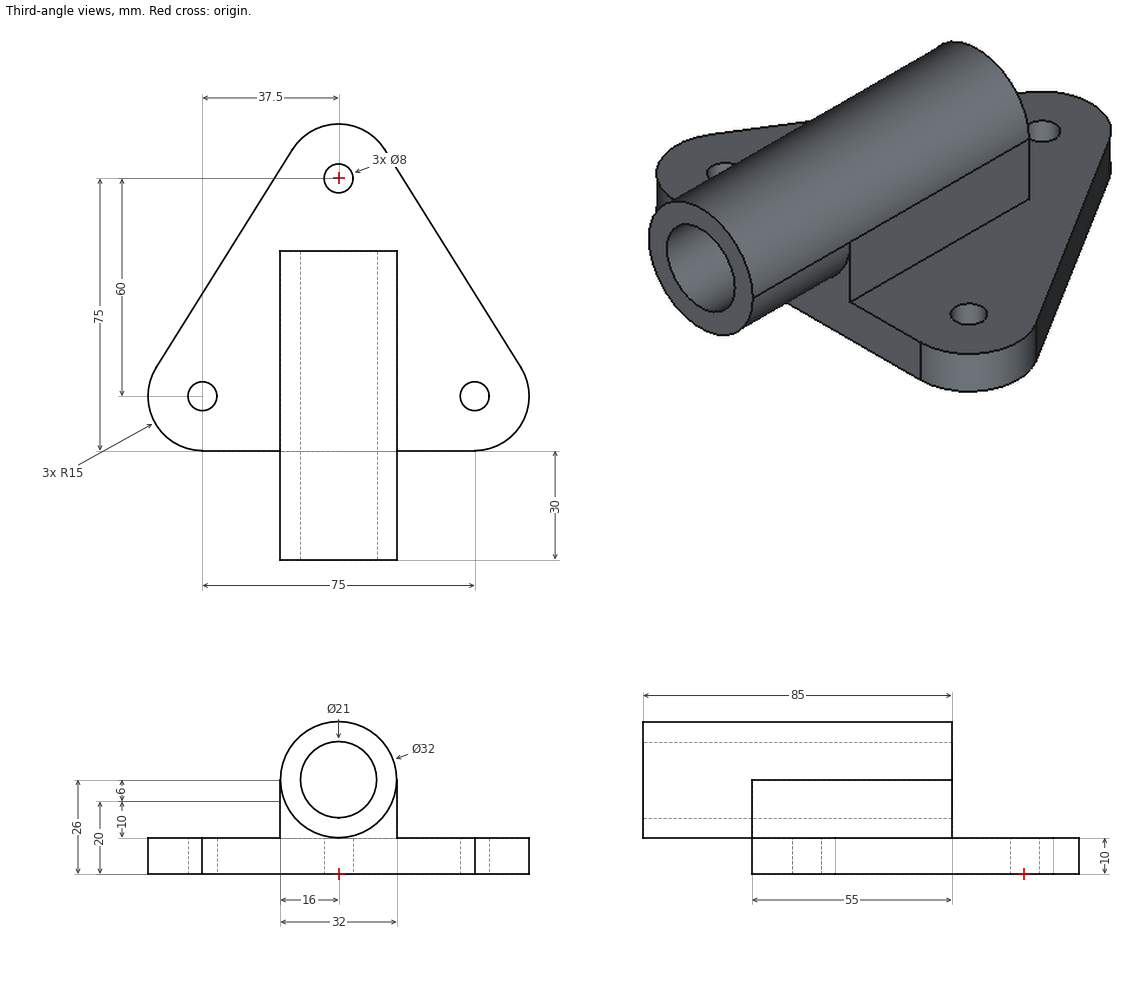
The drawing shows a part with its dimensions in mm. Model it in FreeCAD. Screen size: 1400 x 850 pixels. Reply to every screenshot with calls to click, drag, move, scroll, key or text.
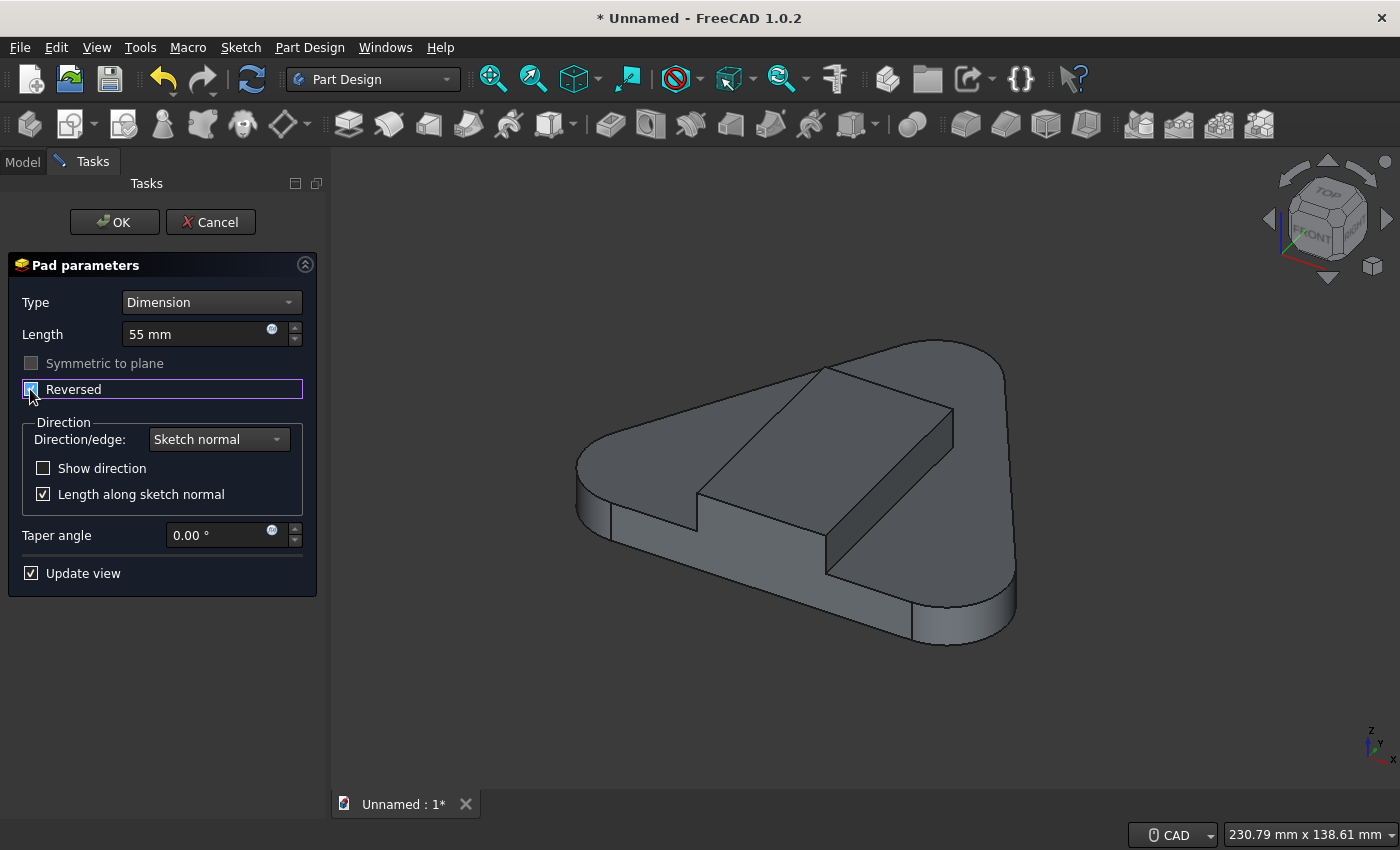
click(115, 222)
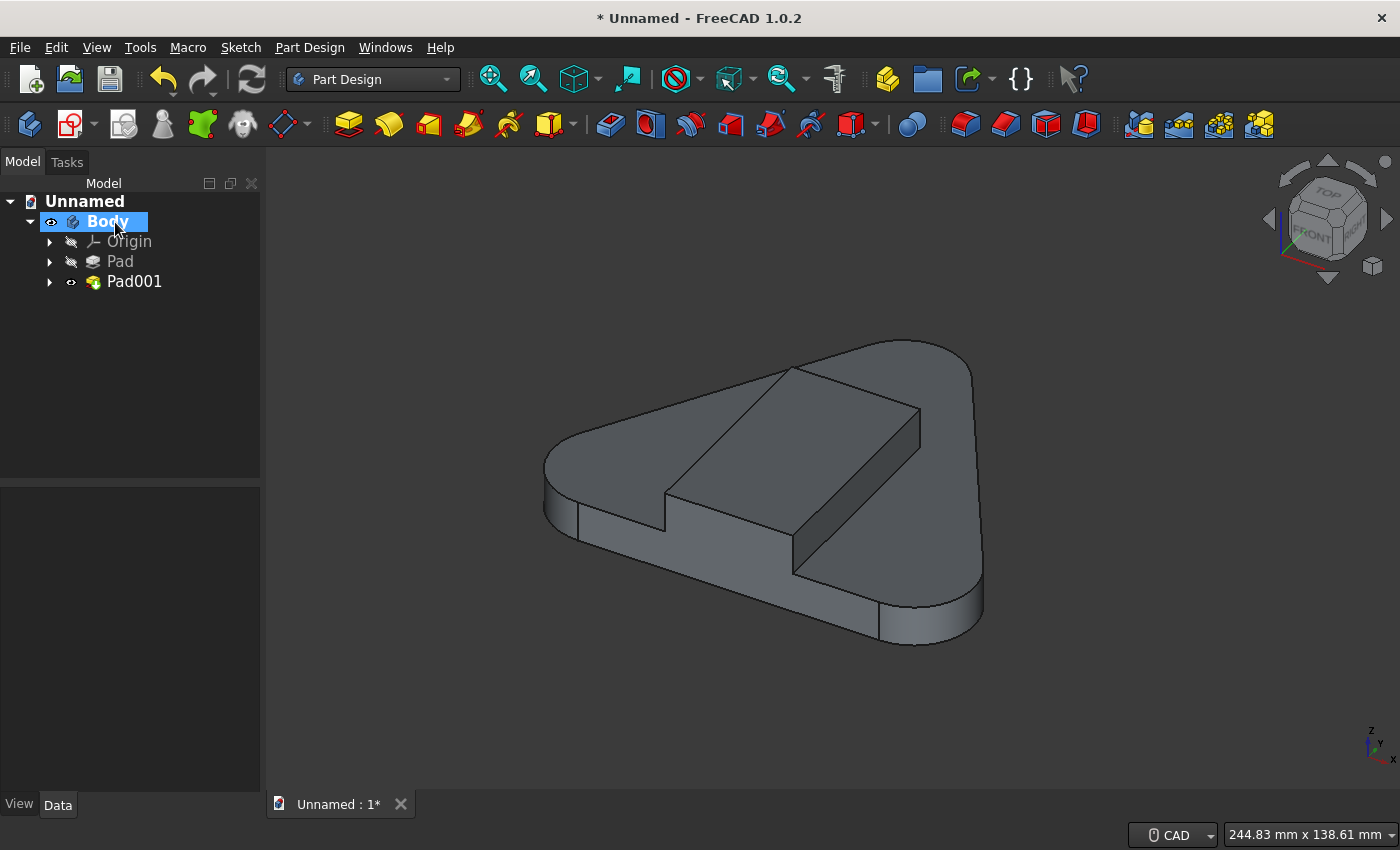
click(729, 551)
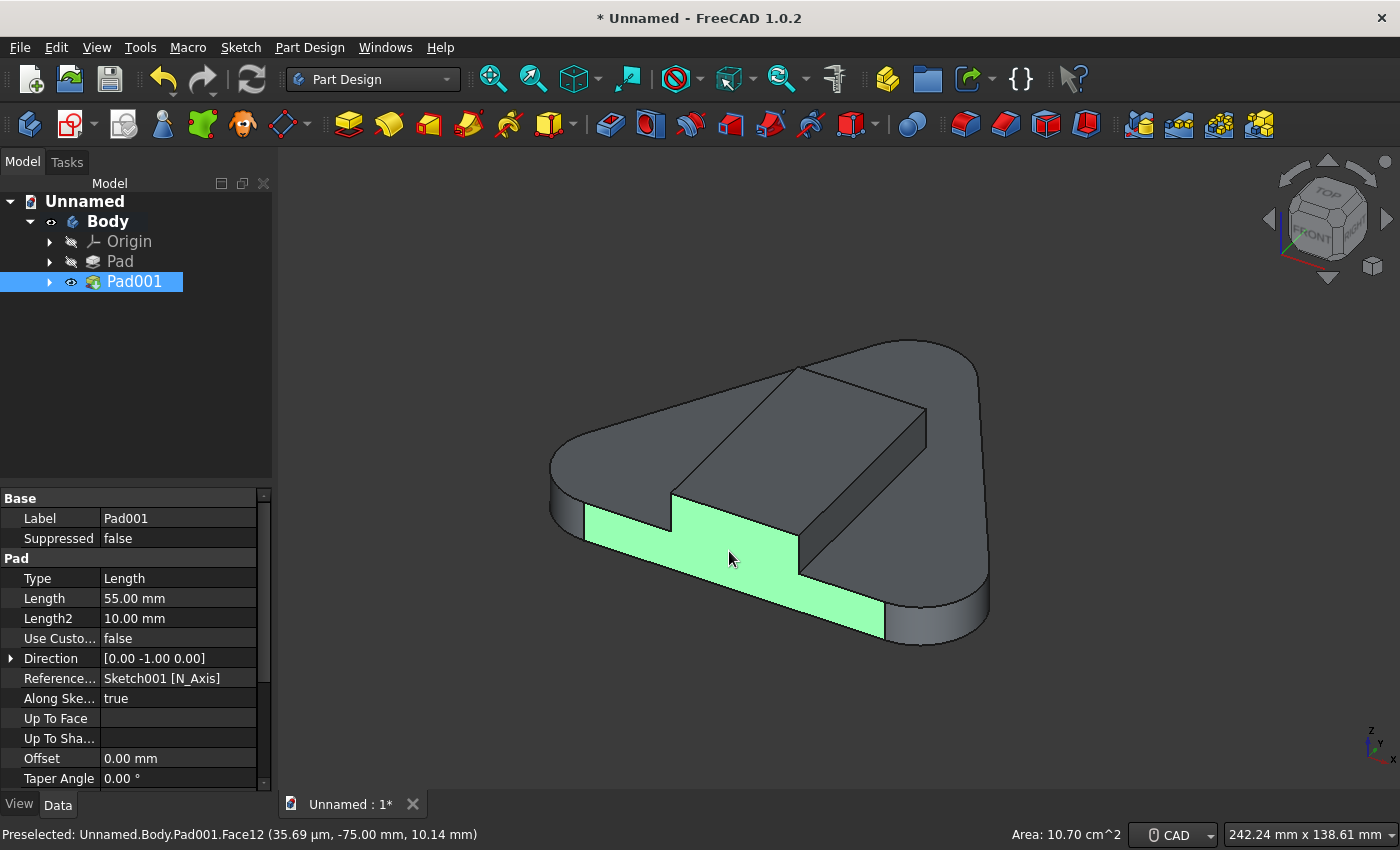
click(70, 124)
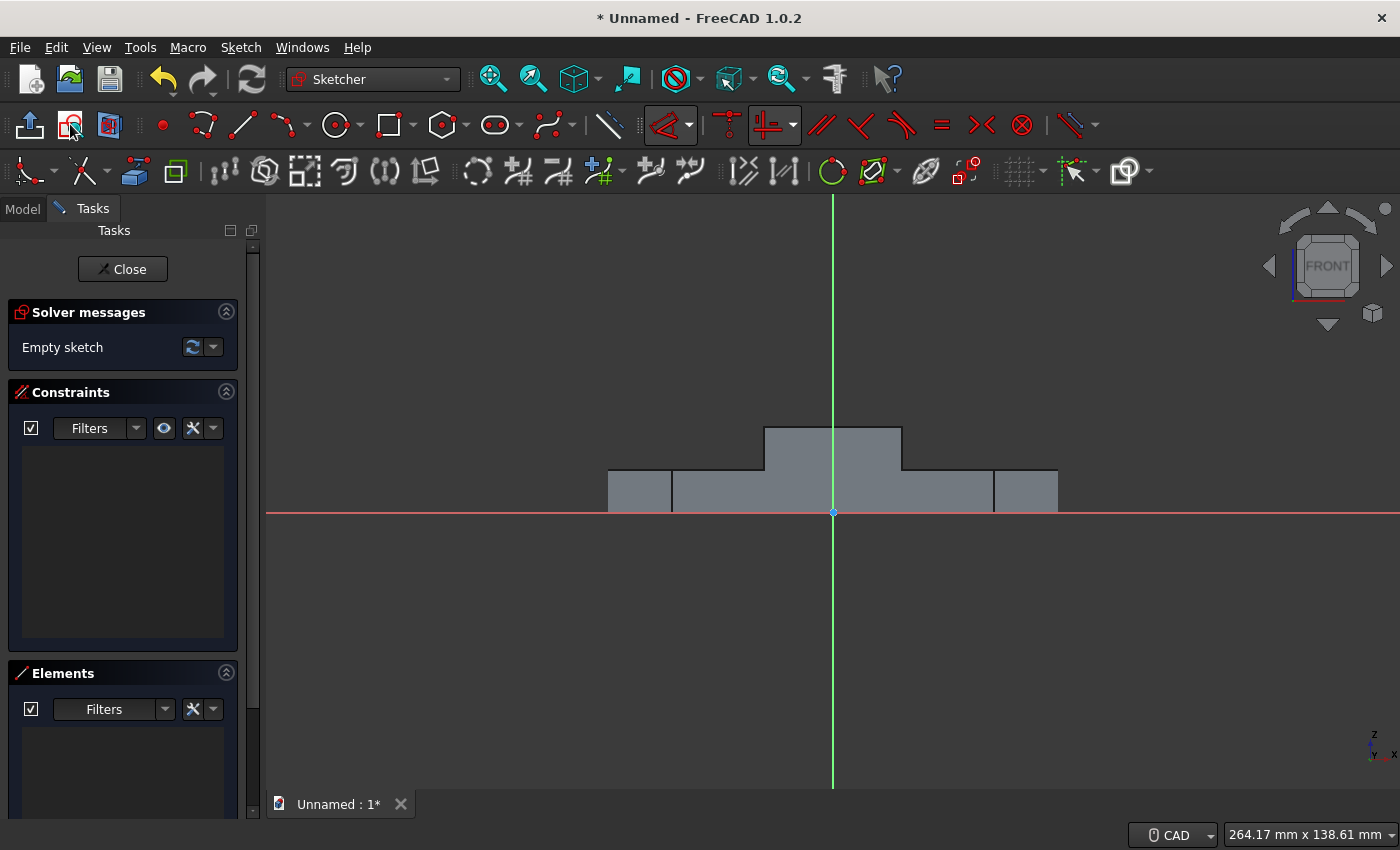
scroll(863, 442, up, 6)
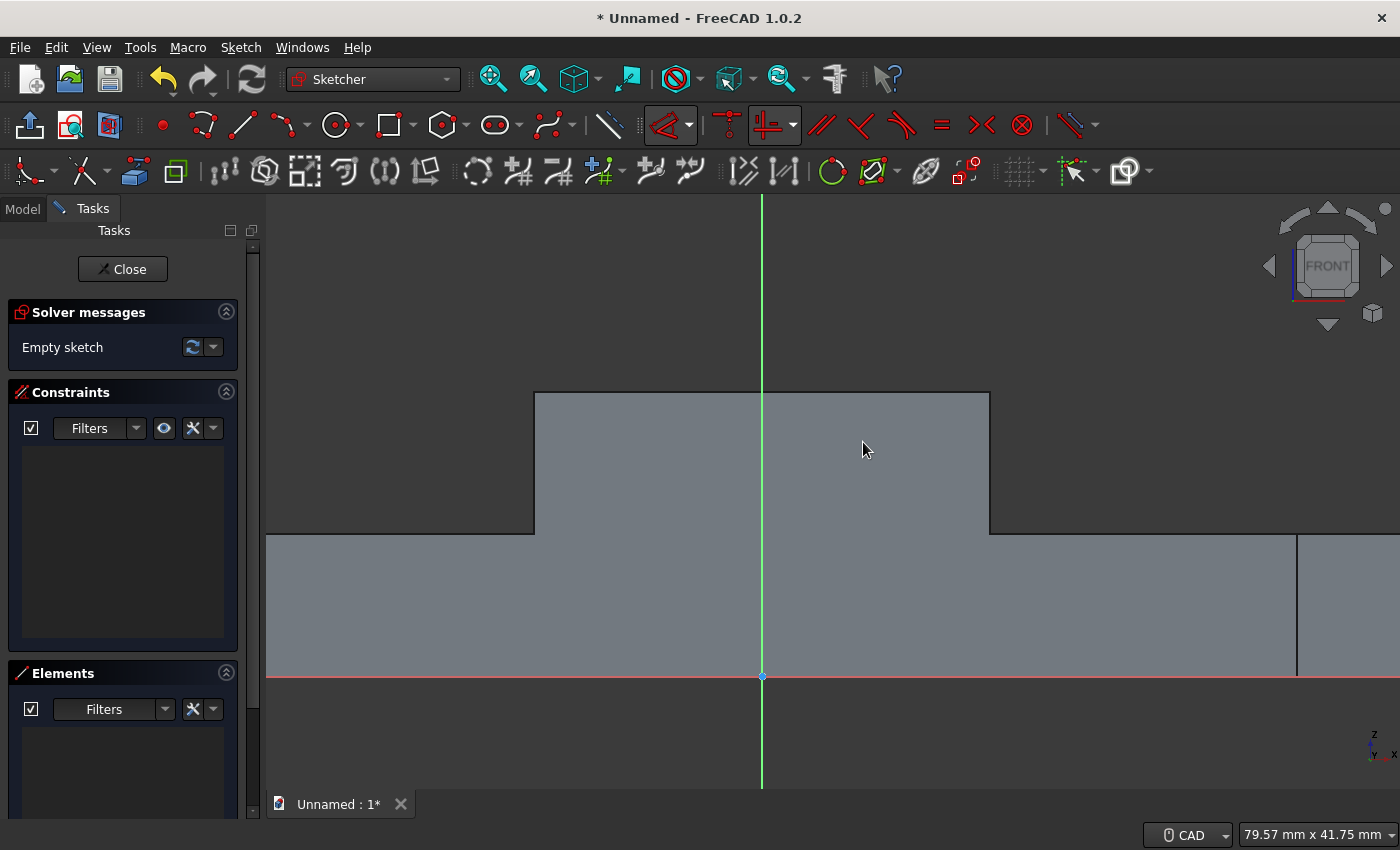
click(390, 126)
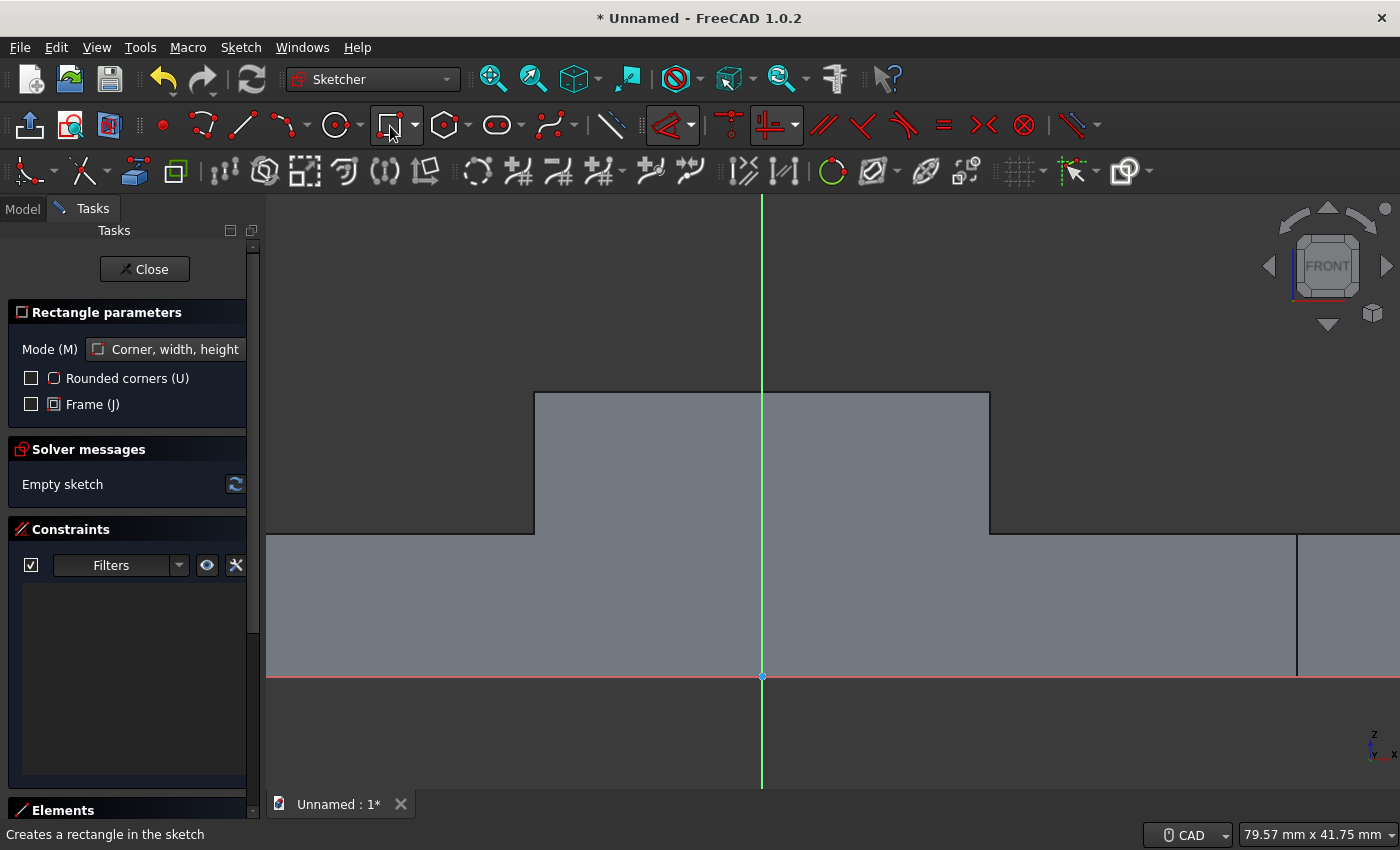
click(534, 306)
click(990, 392)
key(Escape)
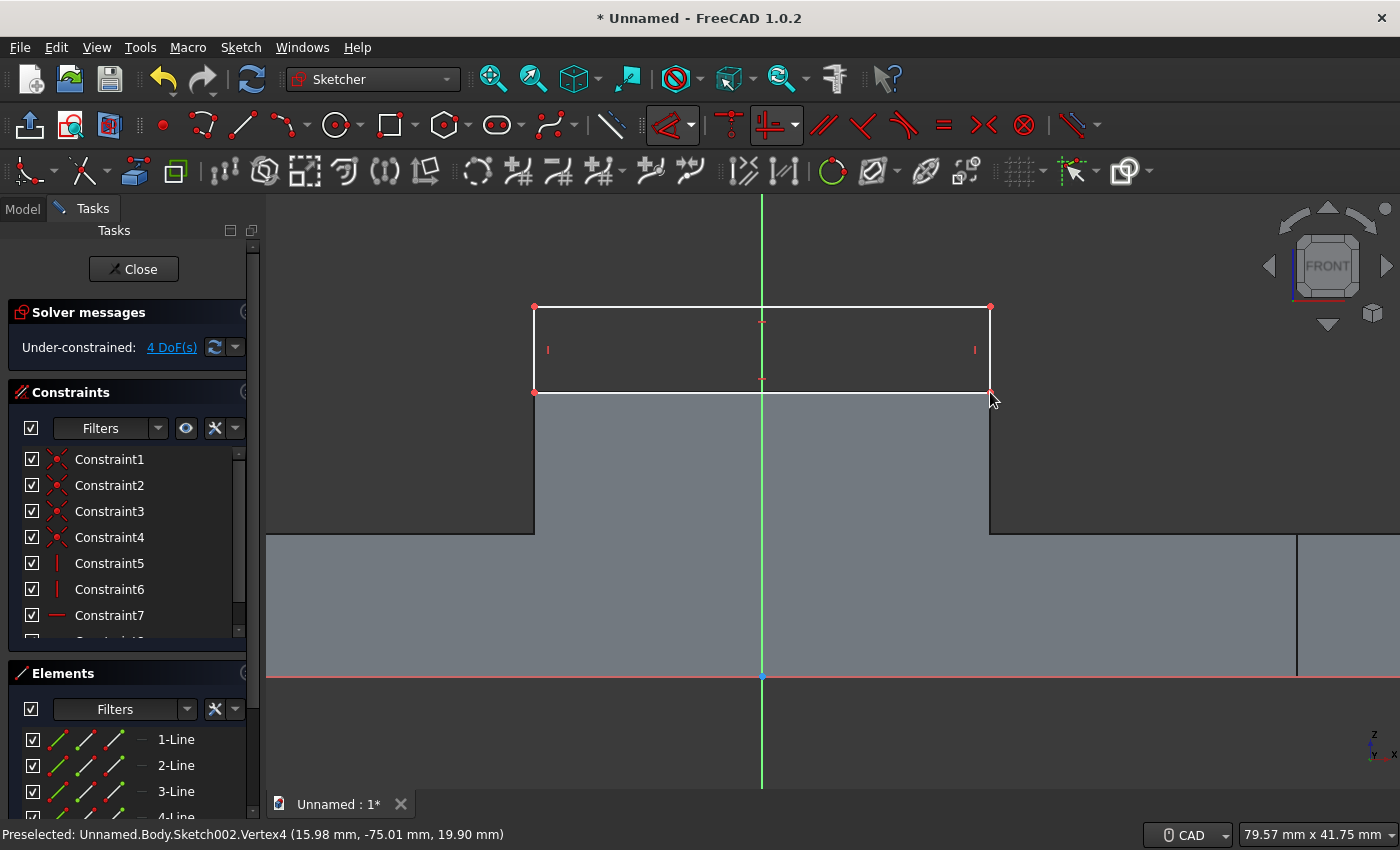
click(534, 333)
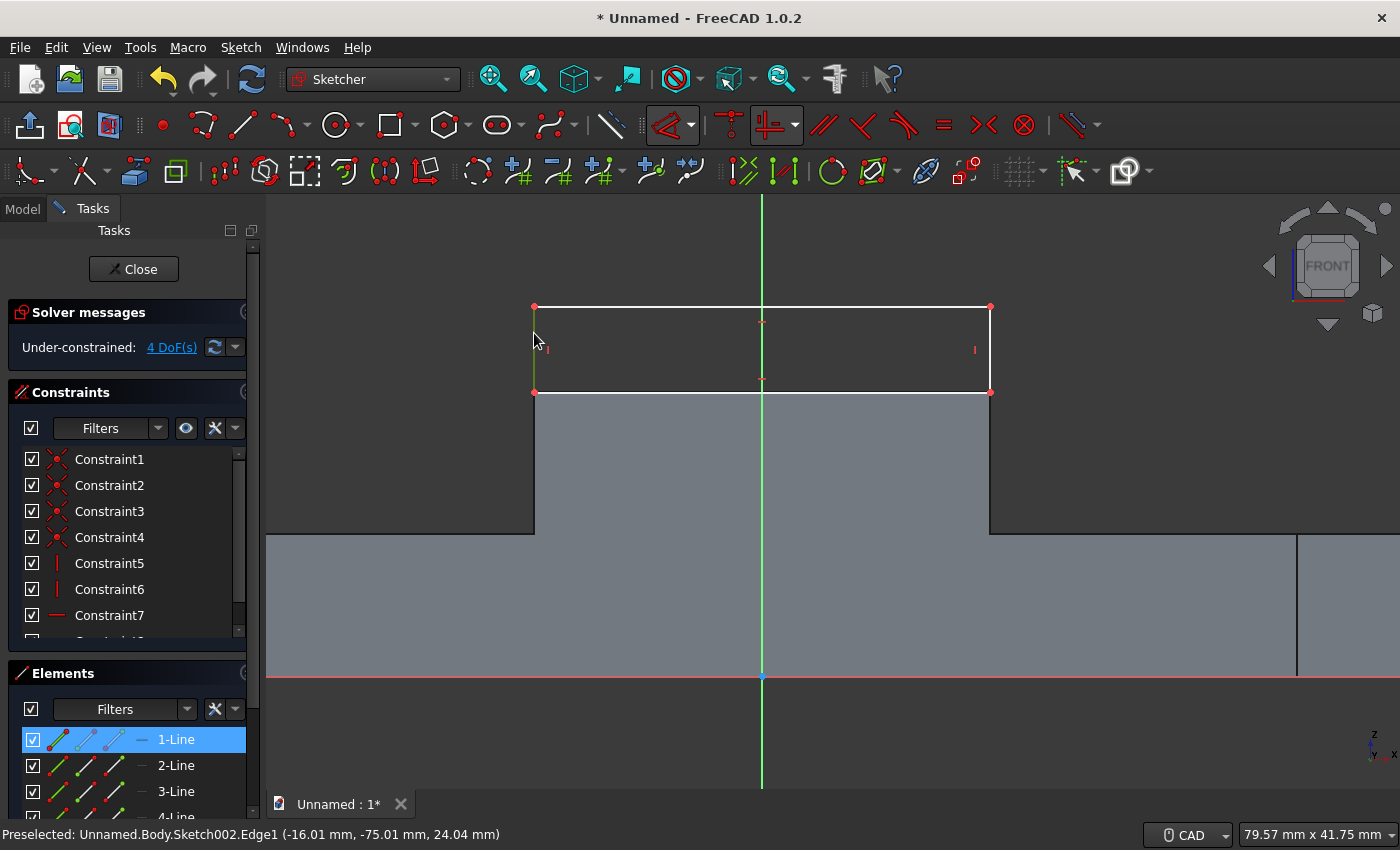
click(694, 126)